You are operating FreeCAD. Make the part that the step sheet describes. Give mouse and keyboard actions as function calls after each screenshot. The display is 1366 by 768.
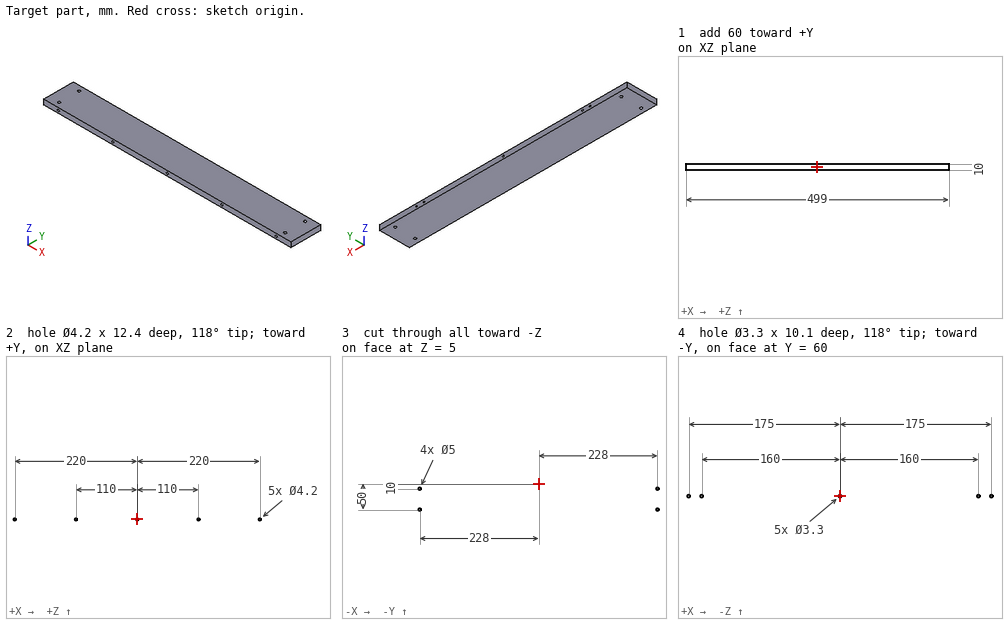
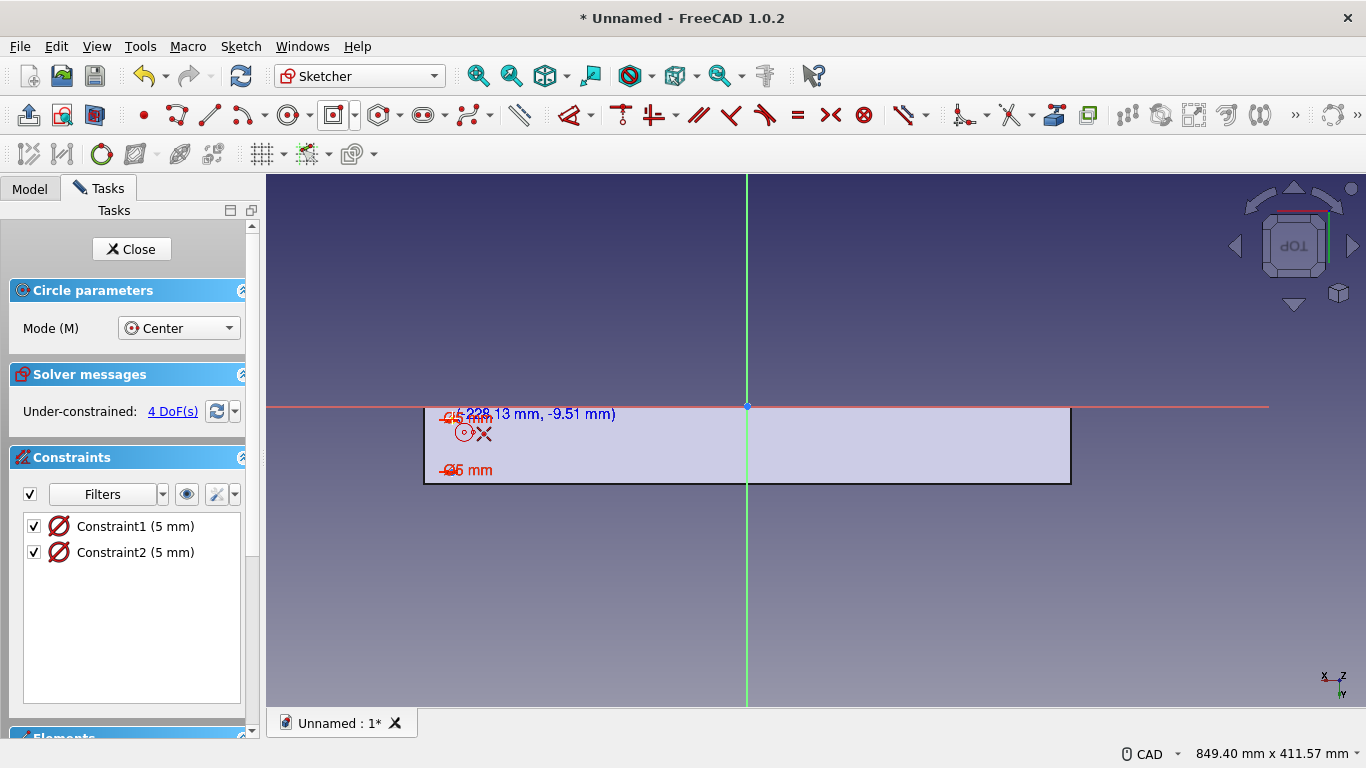
scroll(1043, 419, up, 10)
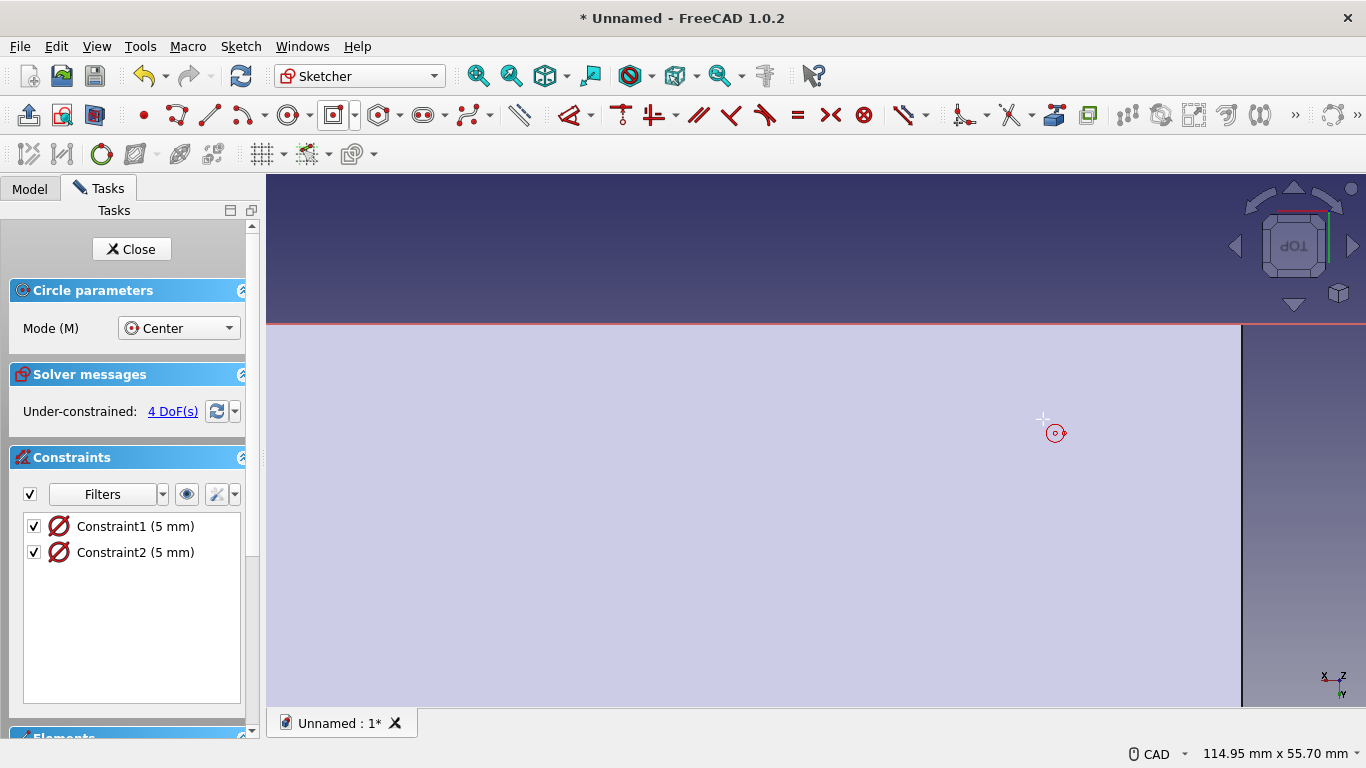
scroll(1044, 419, down, 10)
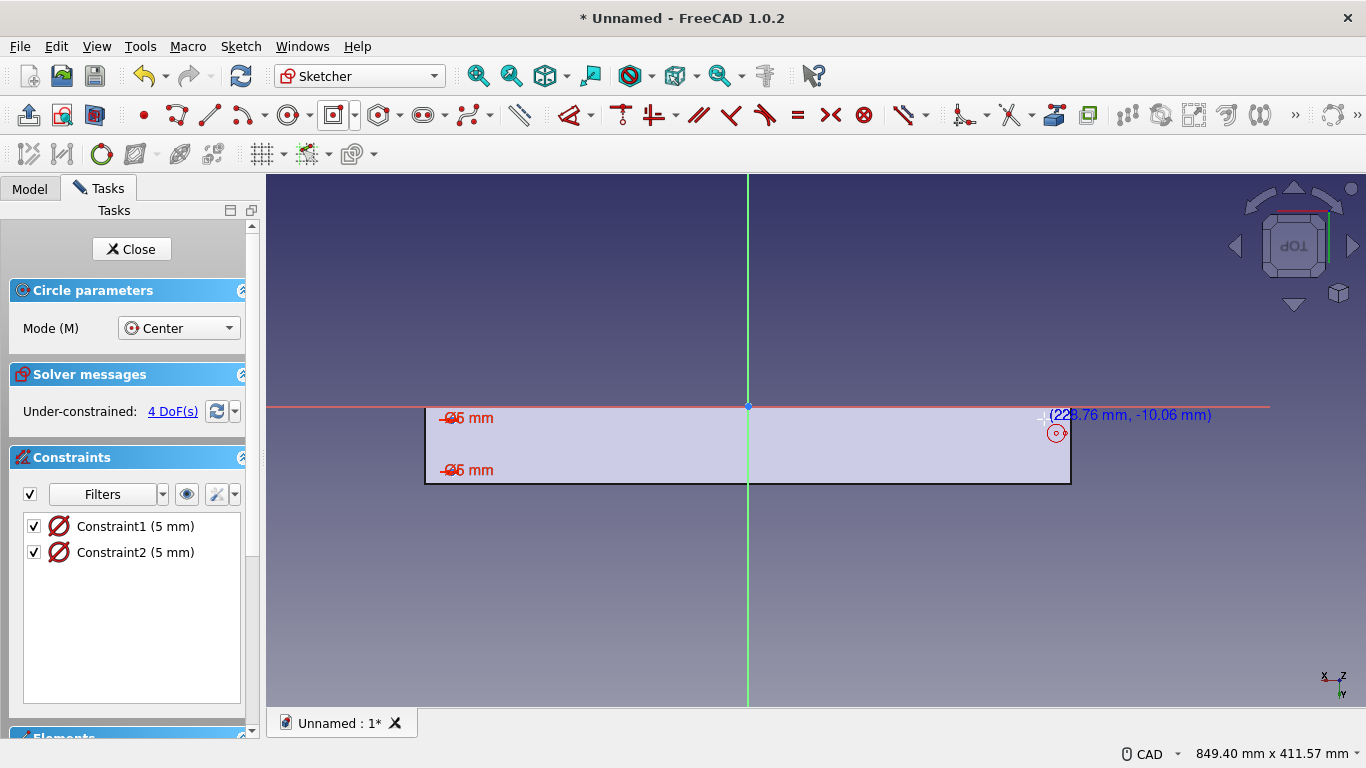
scroll(1044, 419, up, 2)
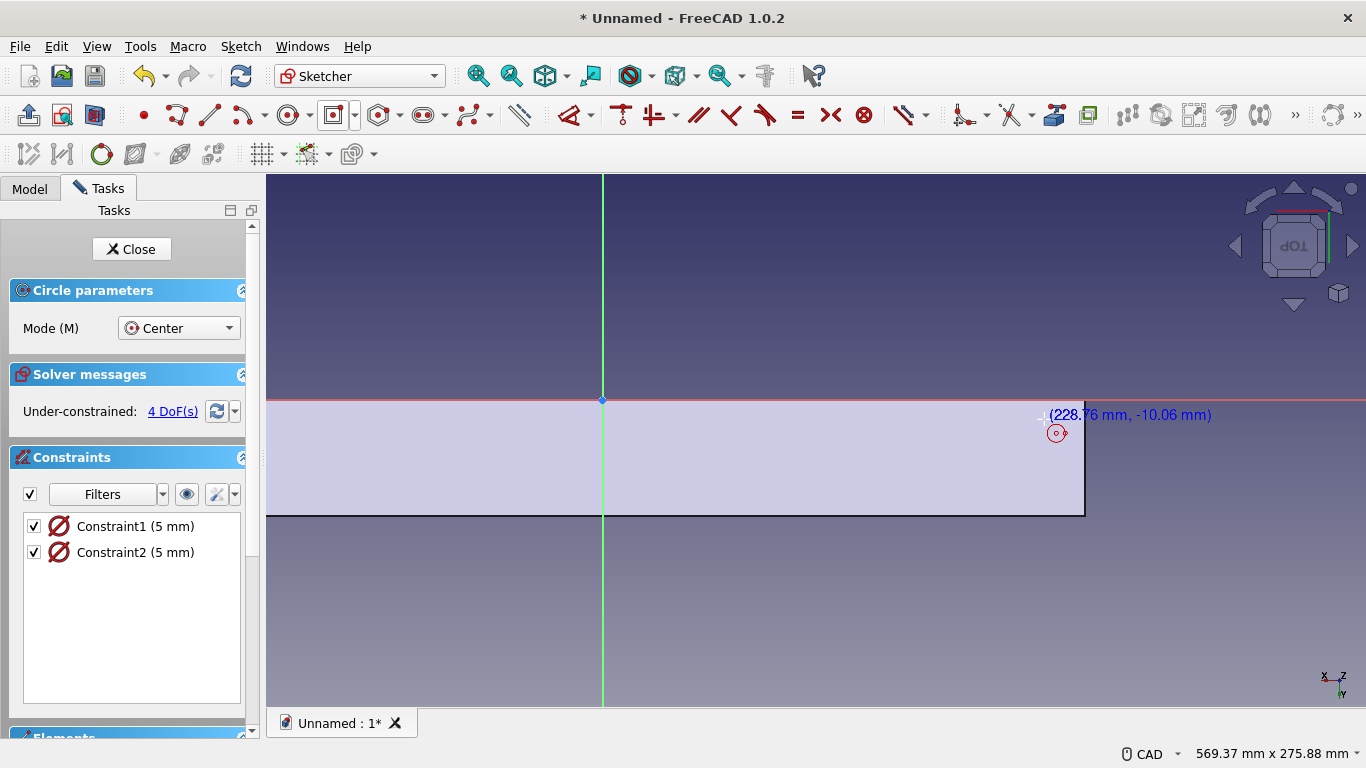
click(1043, 419)
move(1047, 416)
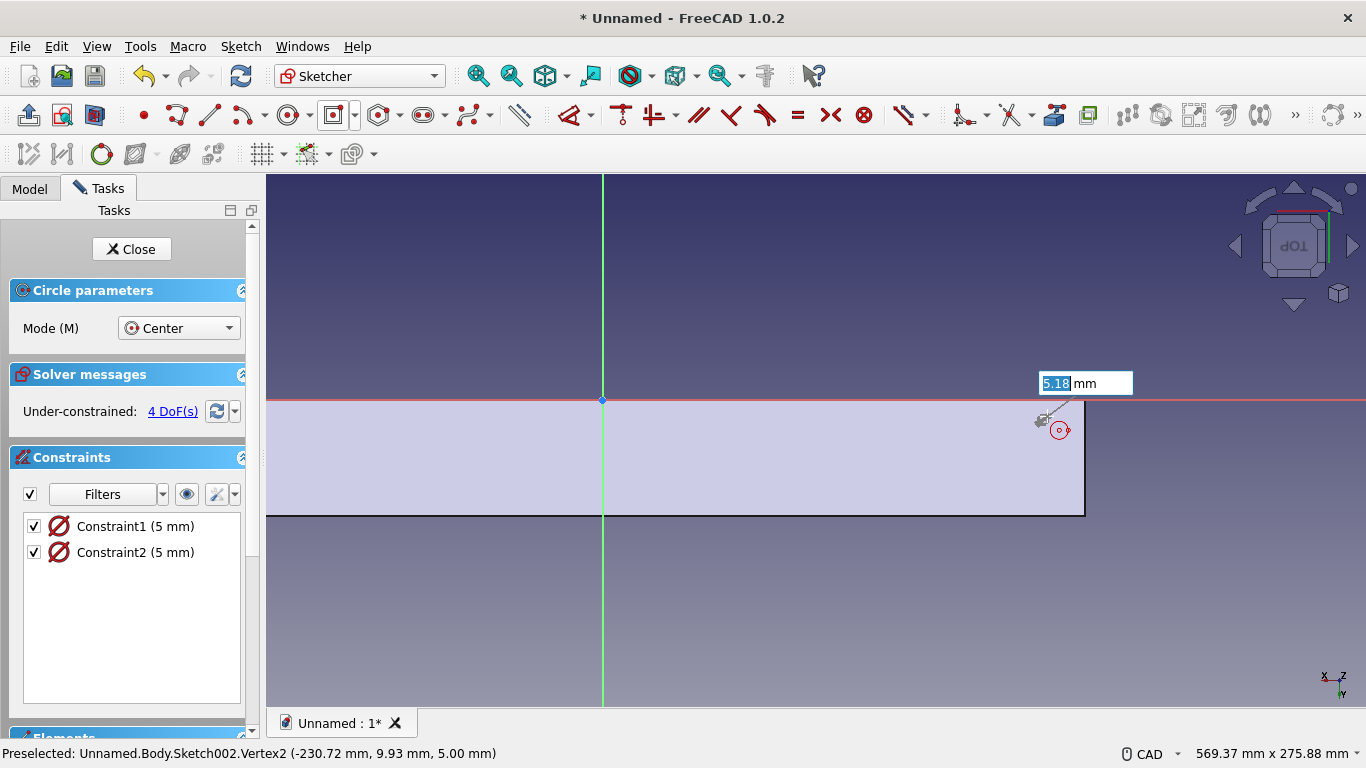
text(5)
key(Return)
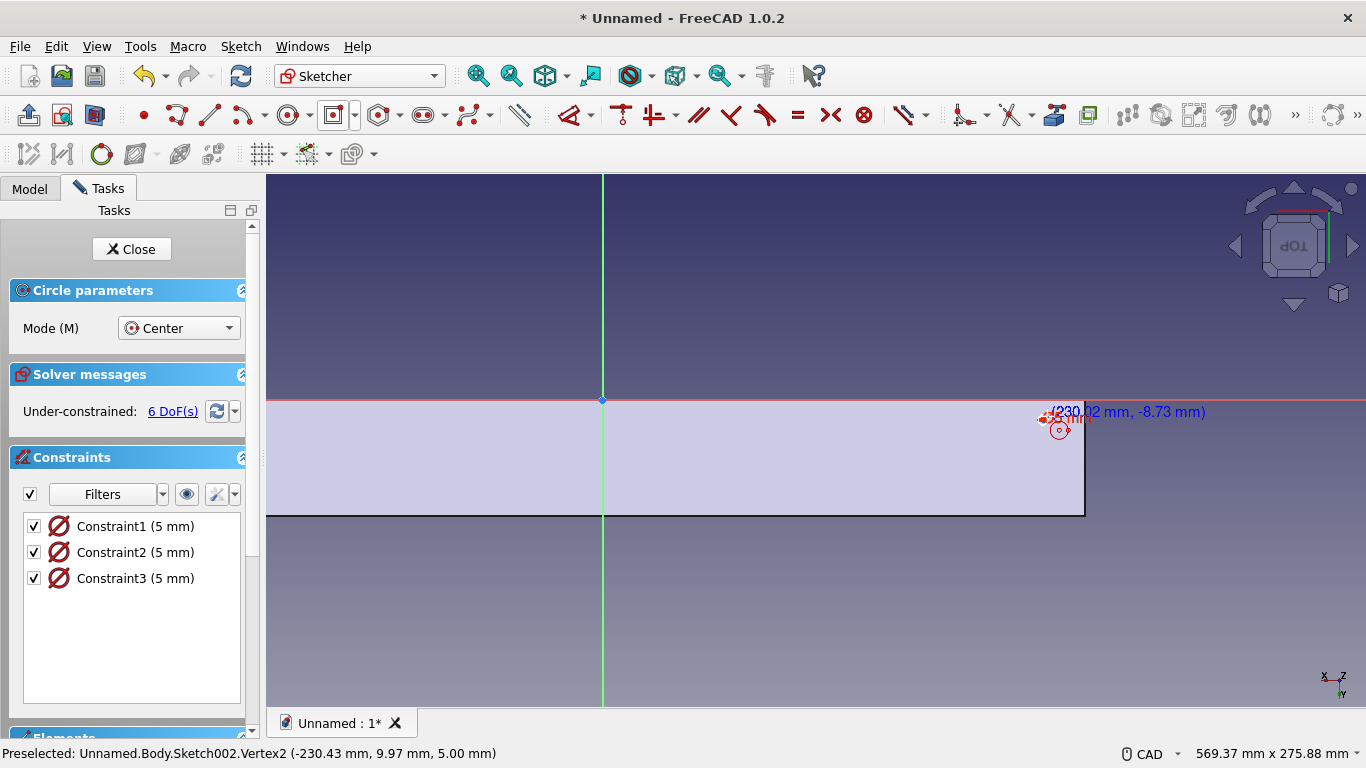
scroll(1043, 497, up, 8)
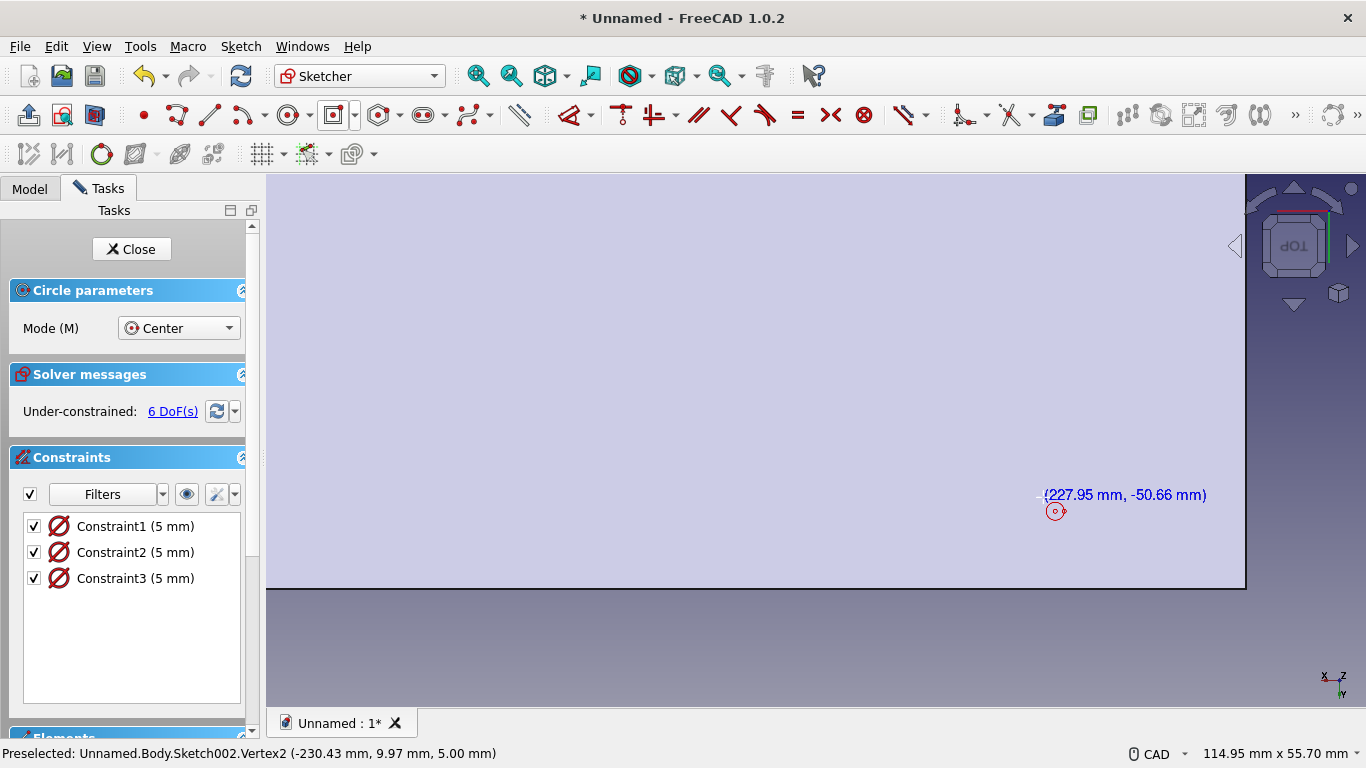
scroll(1043, 468, down, 10)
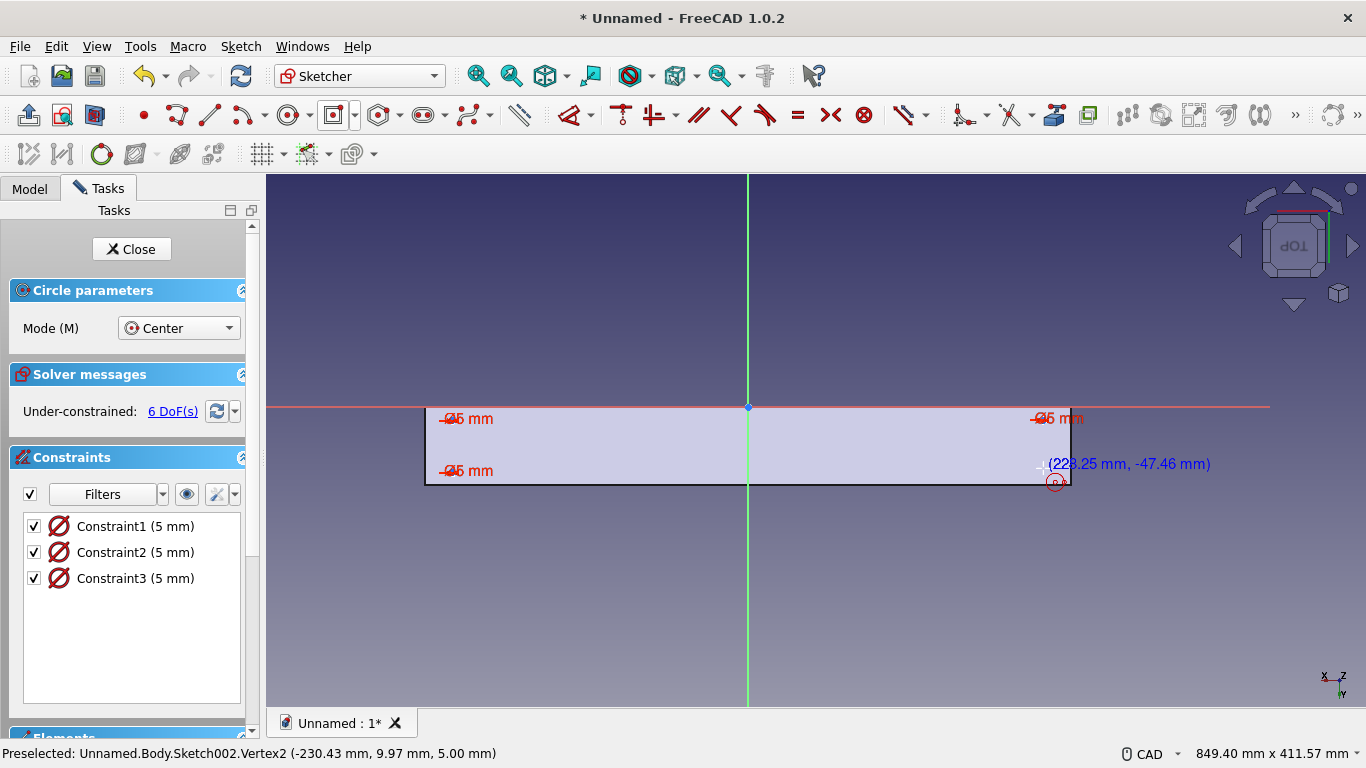
click(1043, 472)
move(1046, 470)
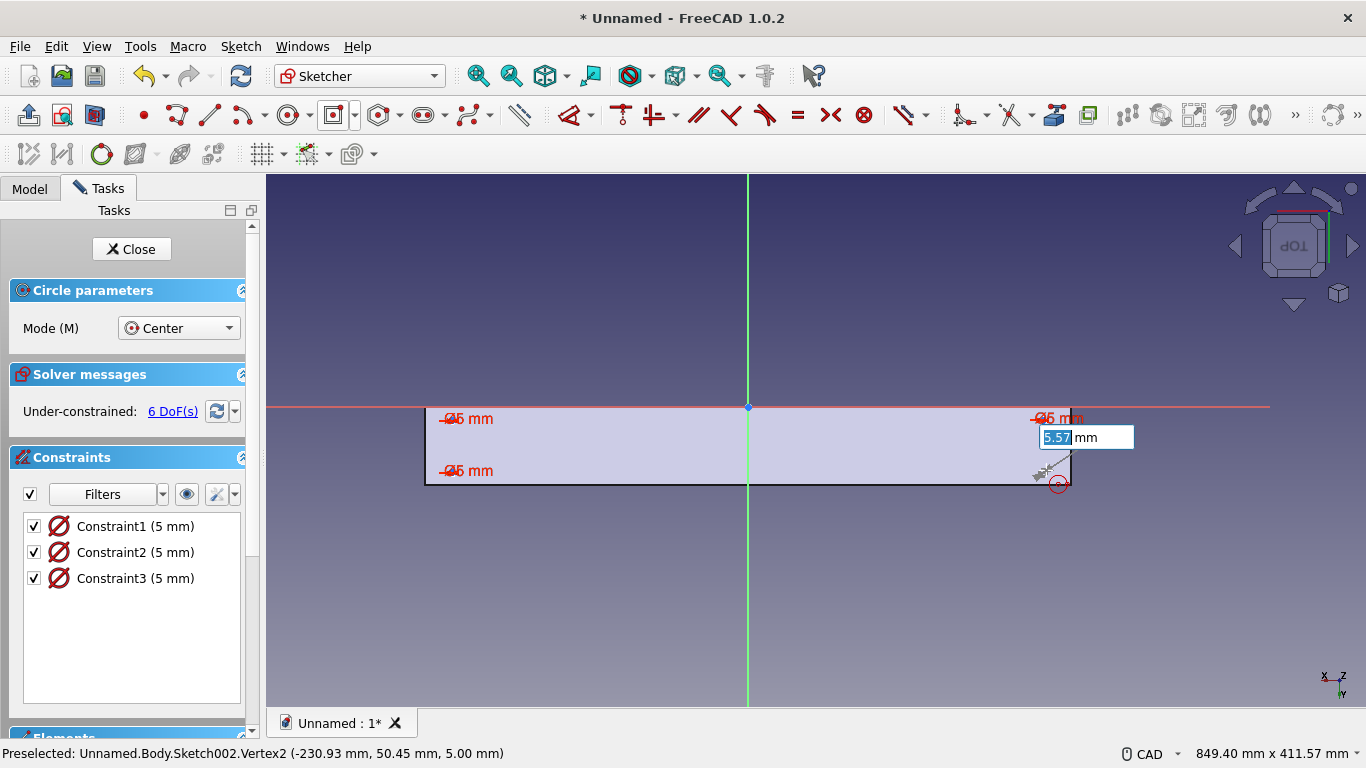
text(5)
key(Return)
key(Escape)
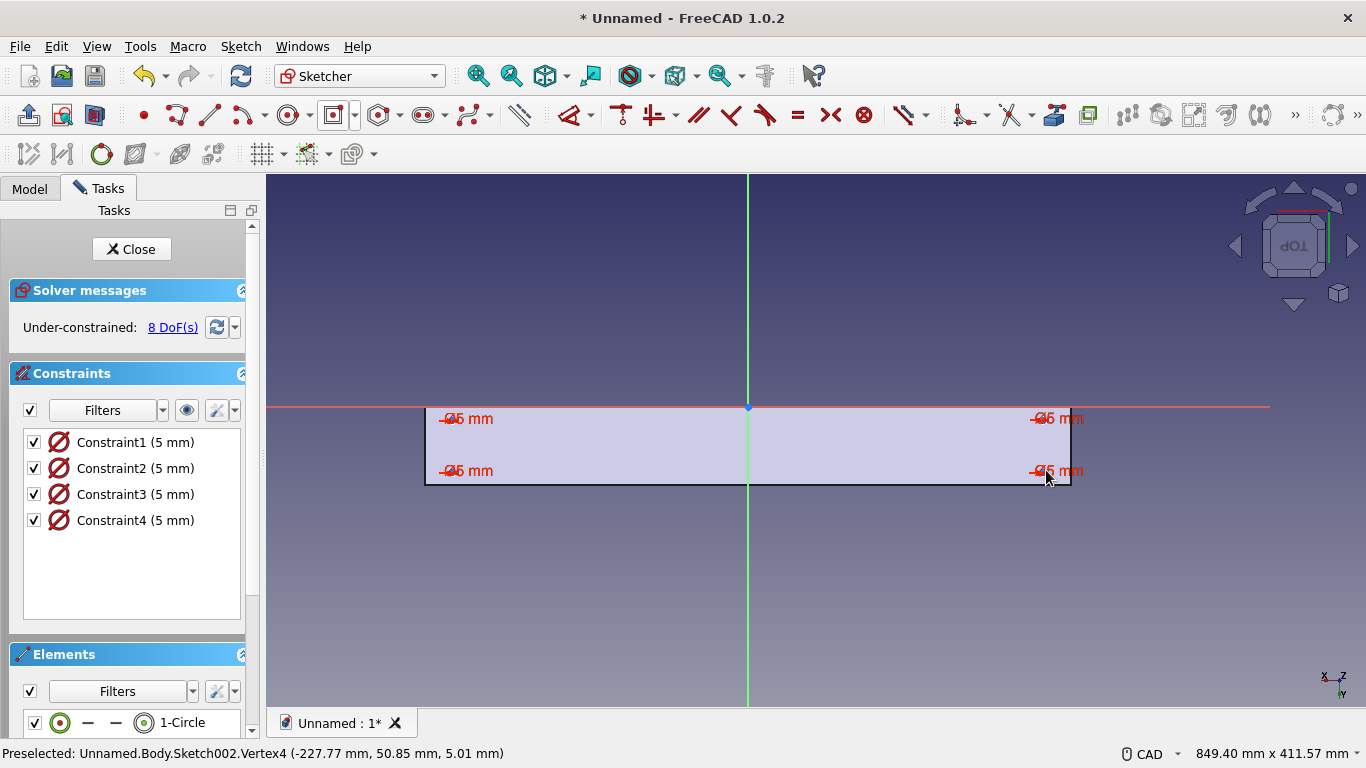
click(453, 473)